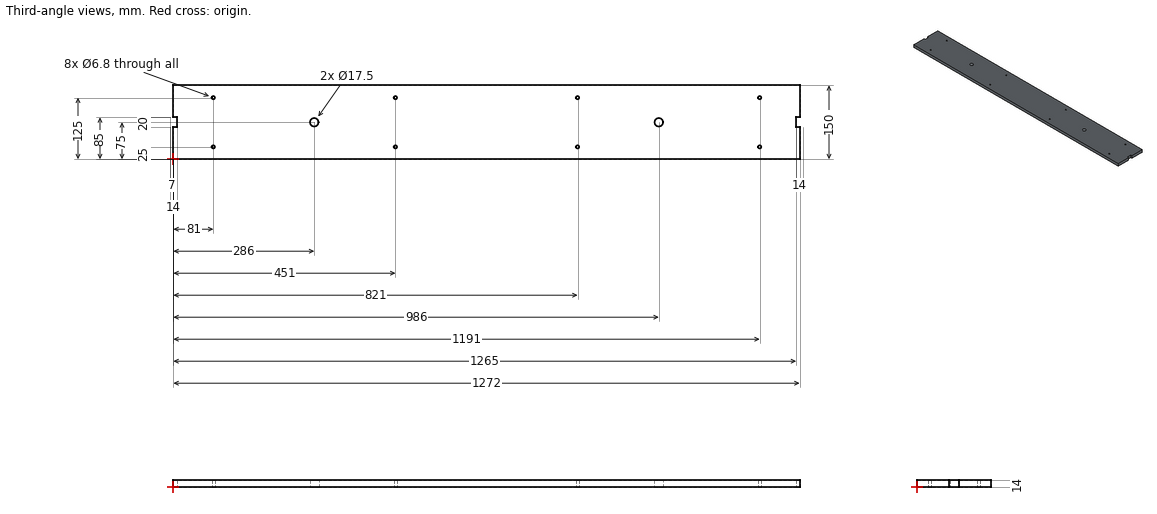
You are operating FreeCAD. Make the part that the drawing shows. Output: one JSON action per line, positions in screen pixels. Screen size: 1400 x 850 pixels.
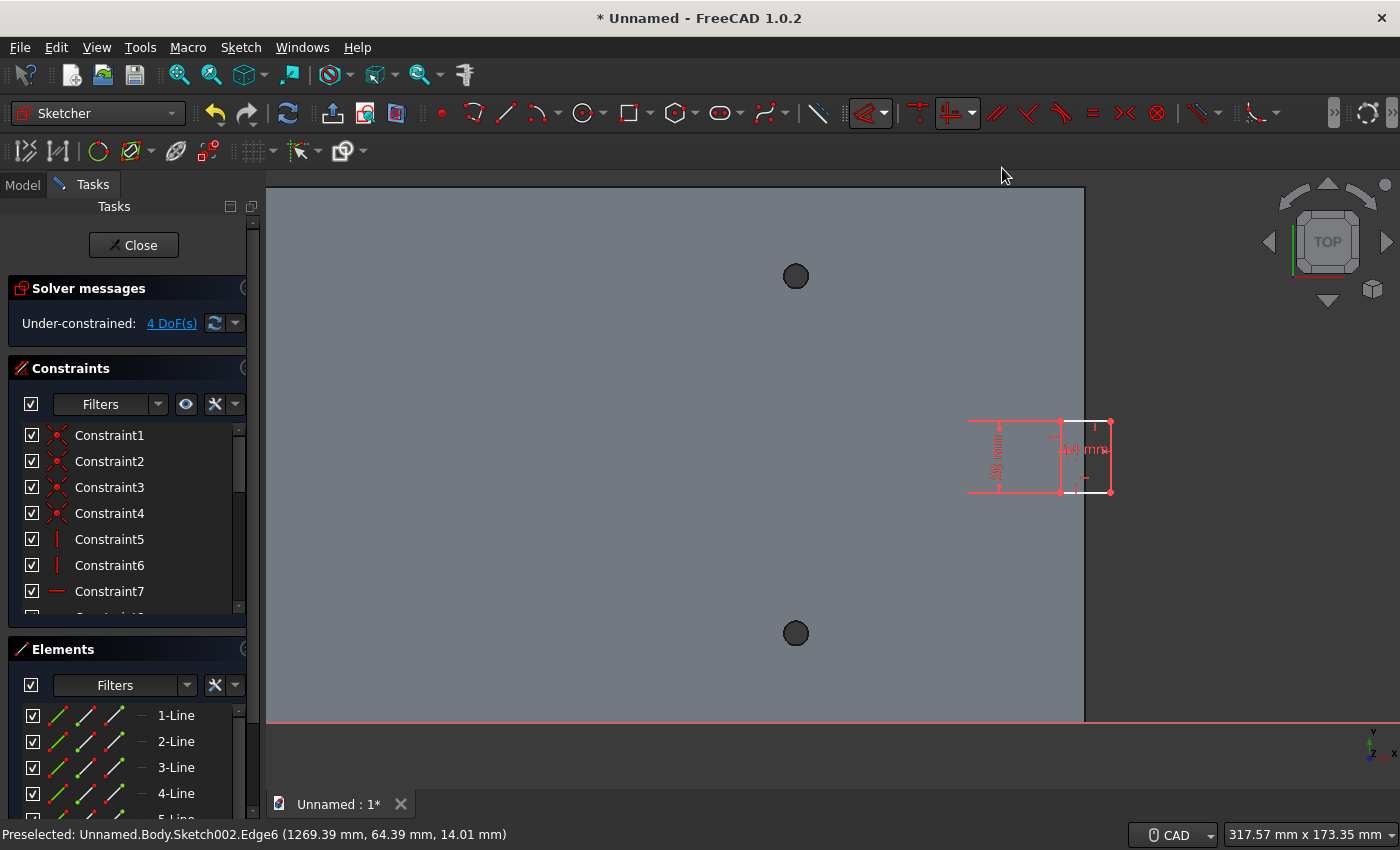
{"action": "scroll", "coordinate": [1070, 465], "scroll_direction": "down", "scroll_amount": 10}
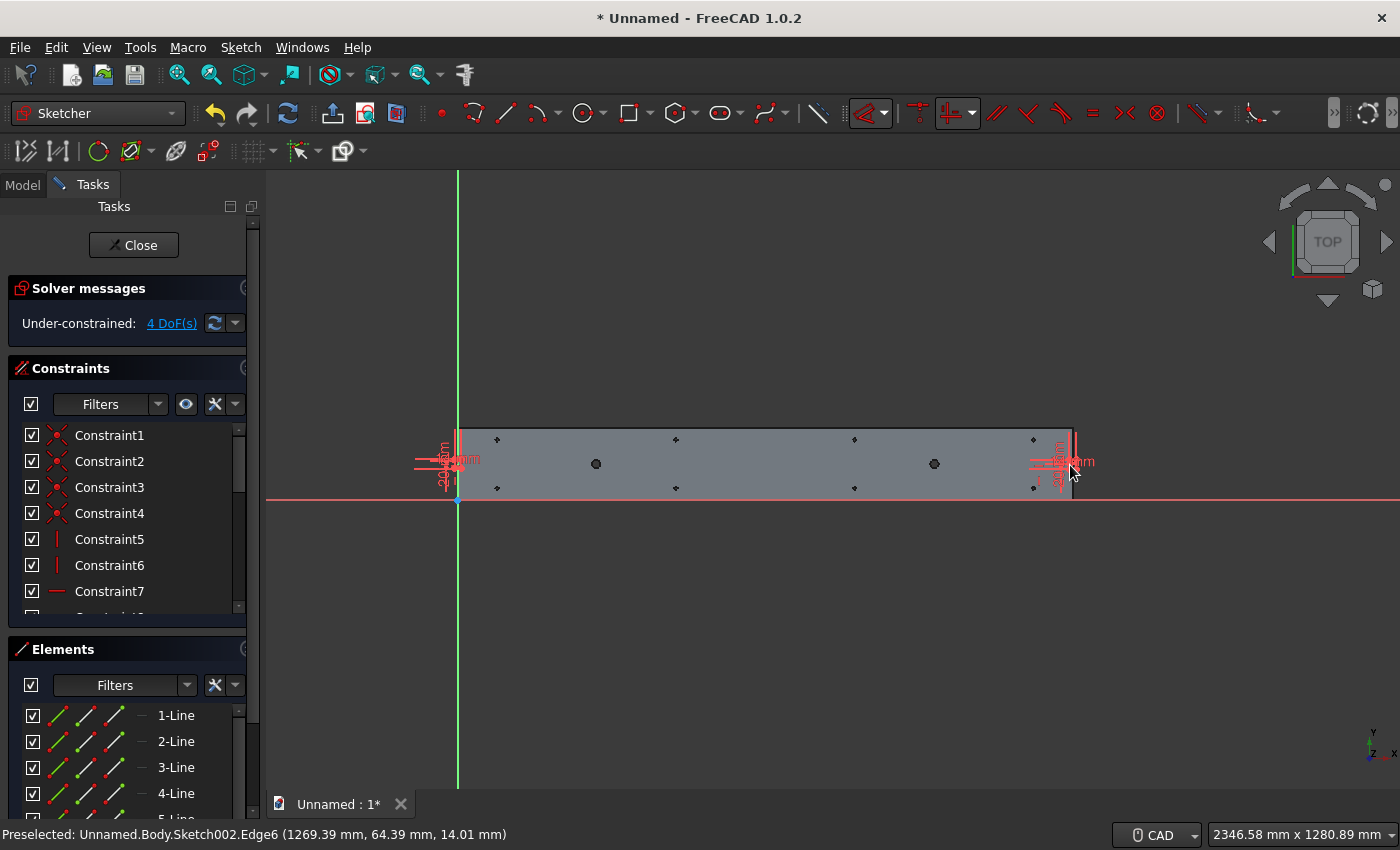
{"action": "scroll", "coordinate": [455, 459], "scroll_direction": "up", "scroll_amount": 13}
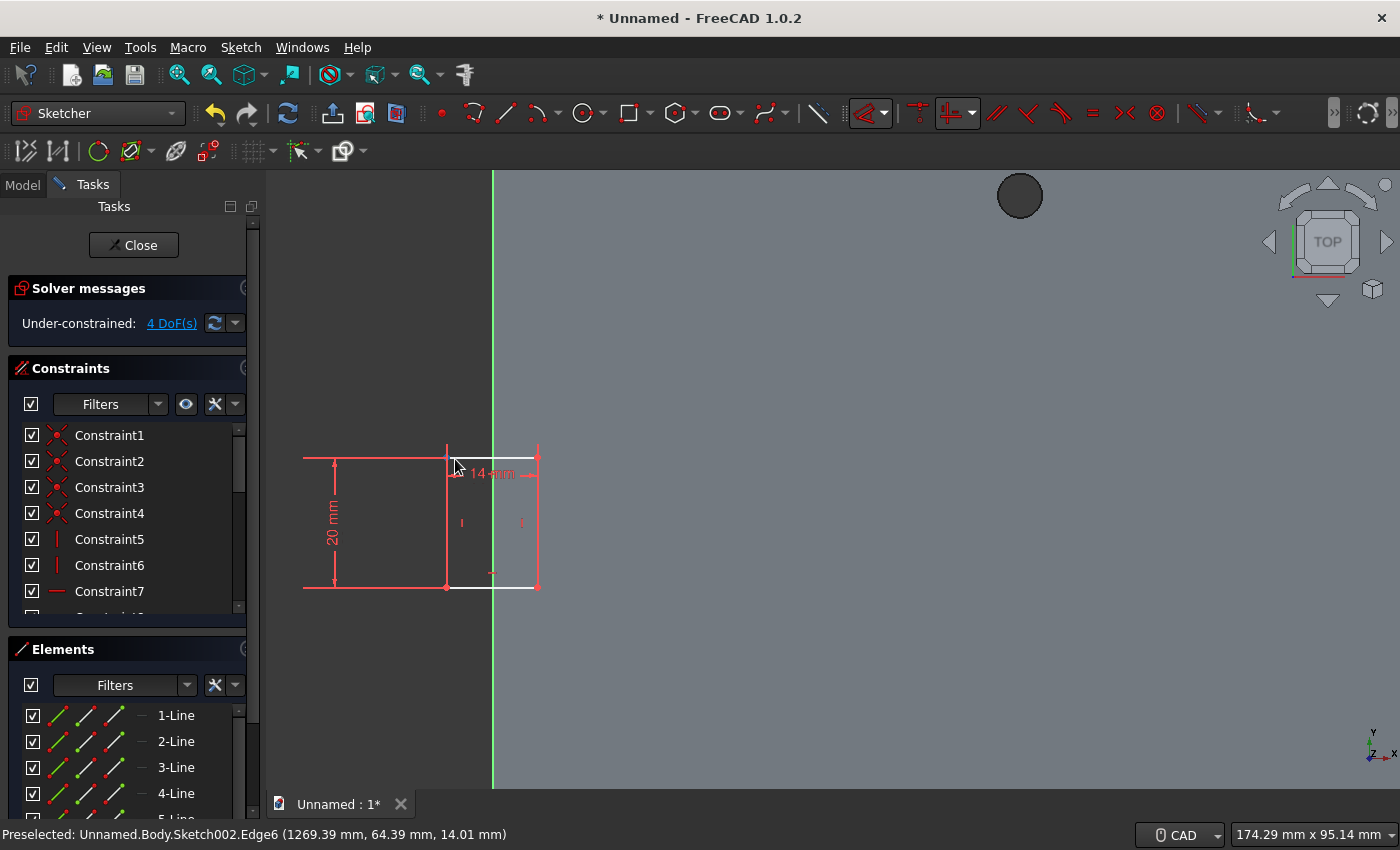
{"action": "left_click", "coordinate": [447, 458]}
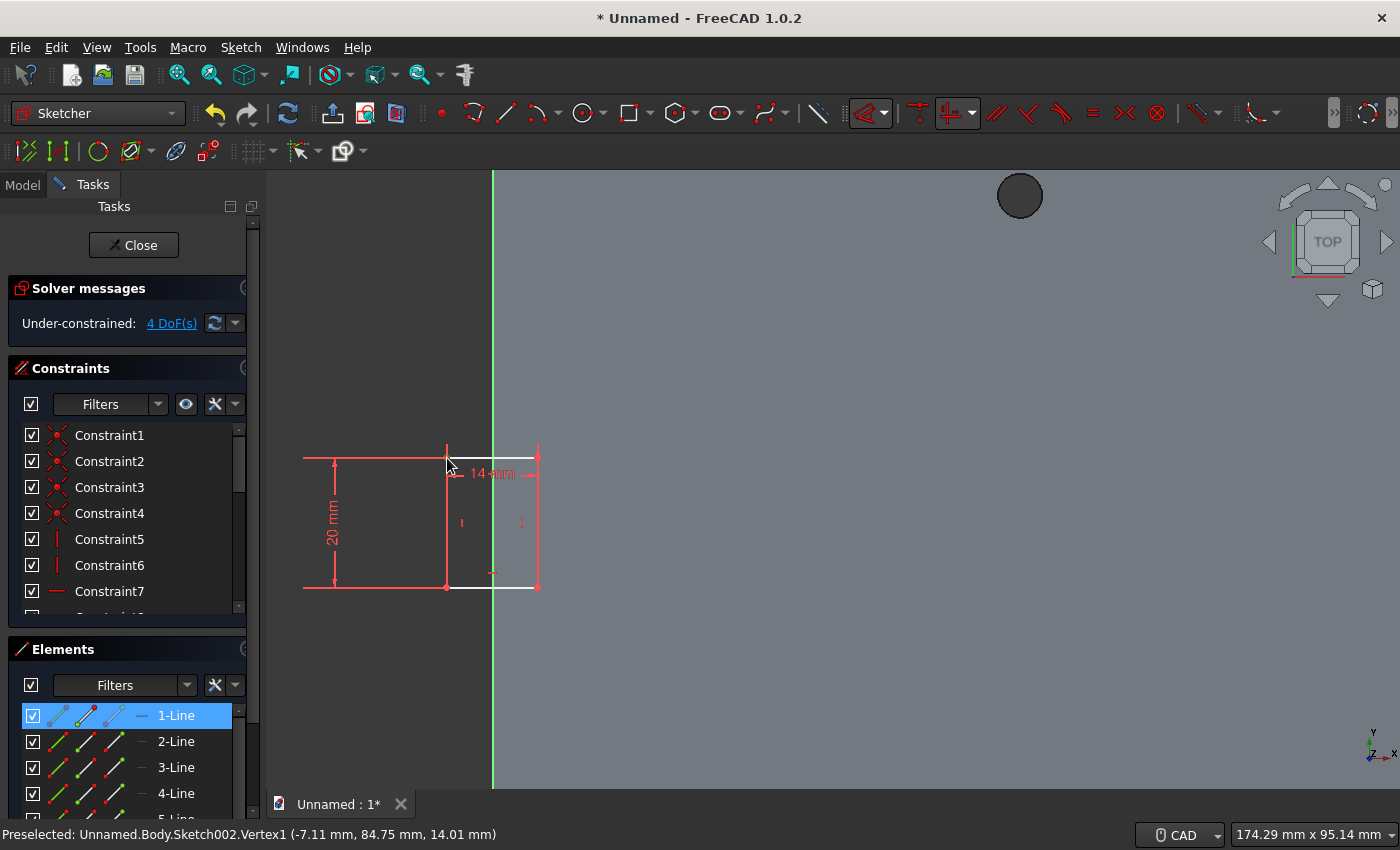
{"action": "key", "text": "l"}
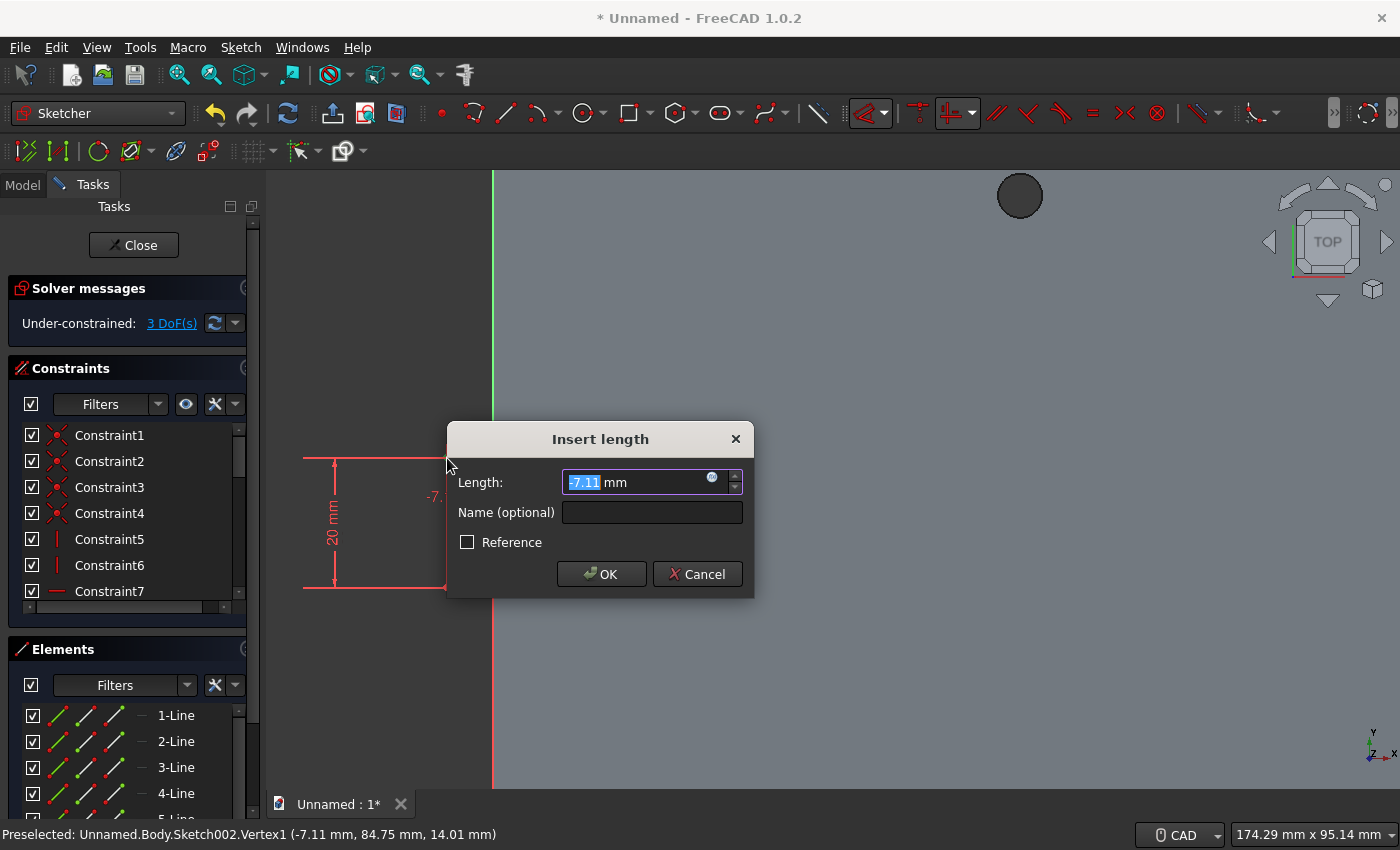
{"action": "type", "text": "-7"}
{"action": "key", "text": "Return"}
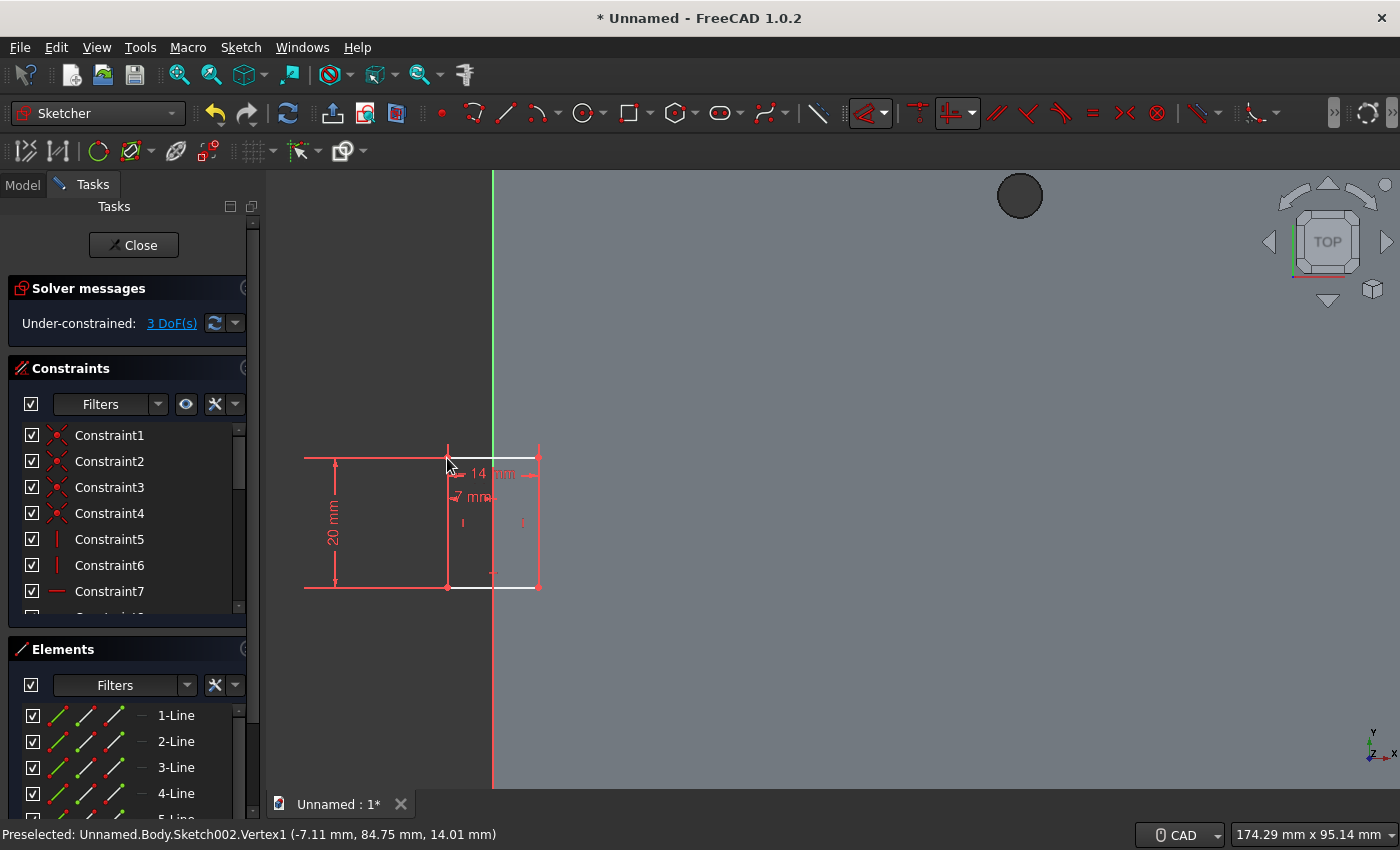
{"action": "scroll", "coordinate": [454, 459], "scroll_direction": "down", "scroll_amount": 13}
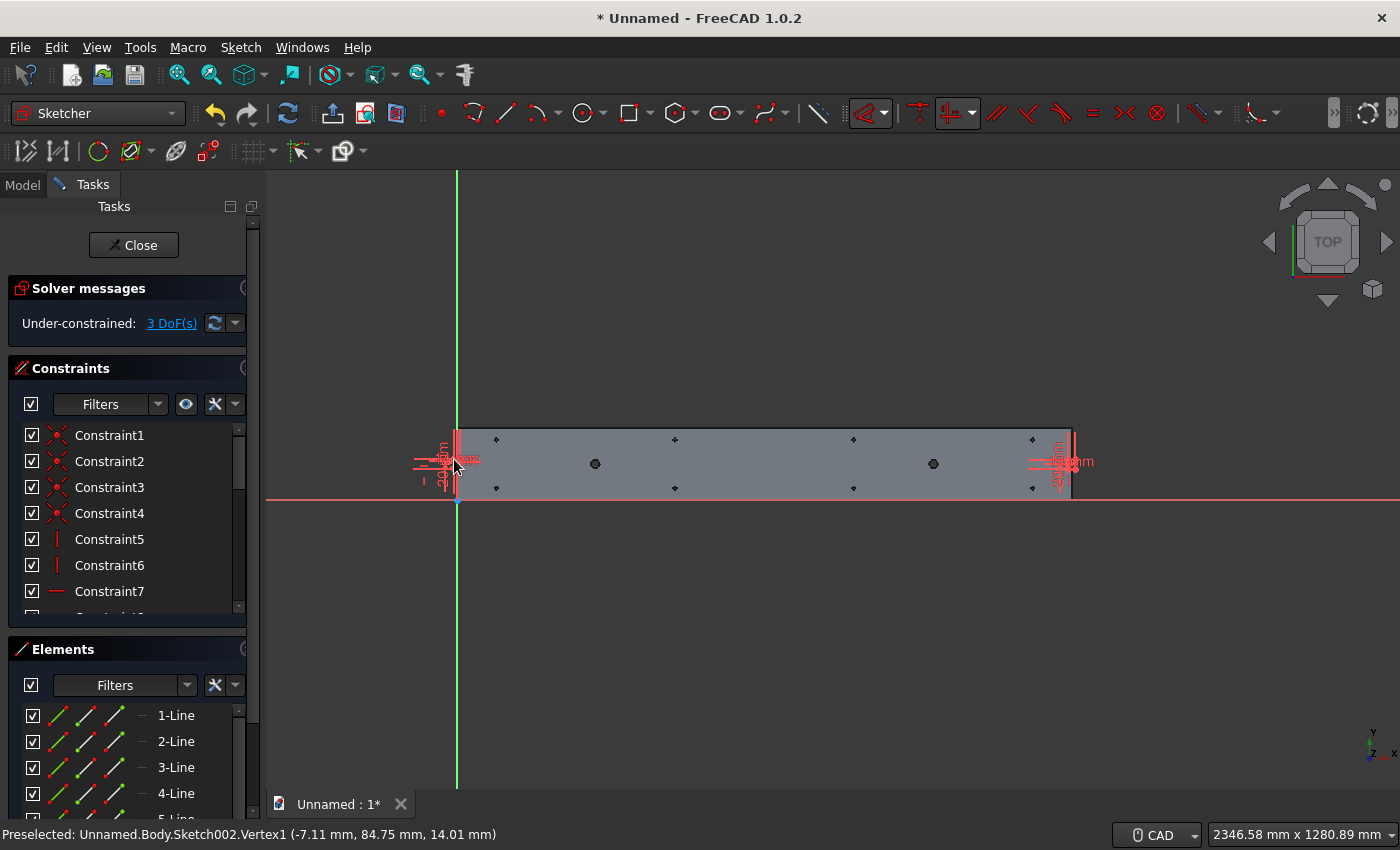
{"action": "scroll", "coordinate": [454, 459], "scroll_direction": "up", "scroll_amount": 3}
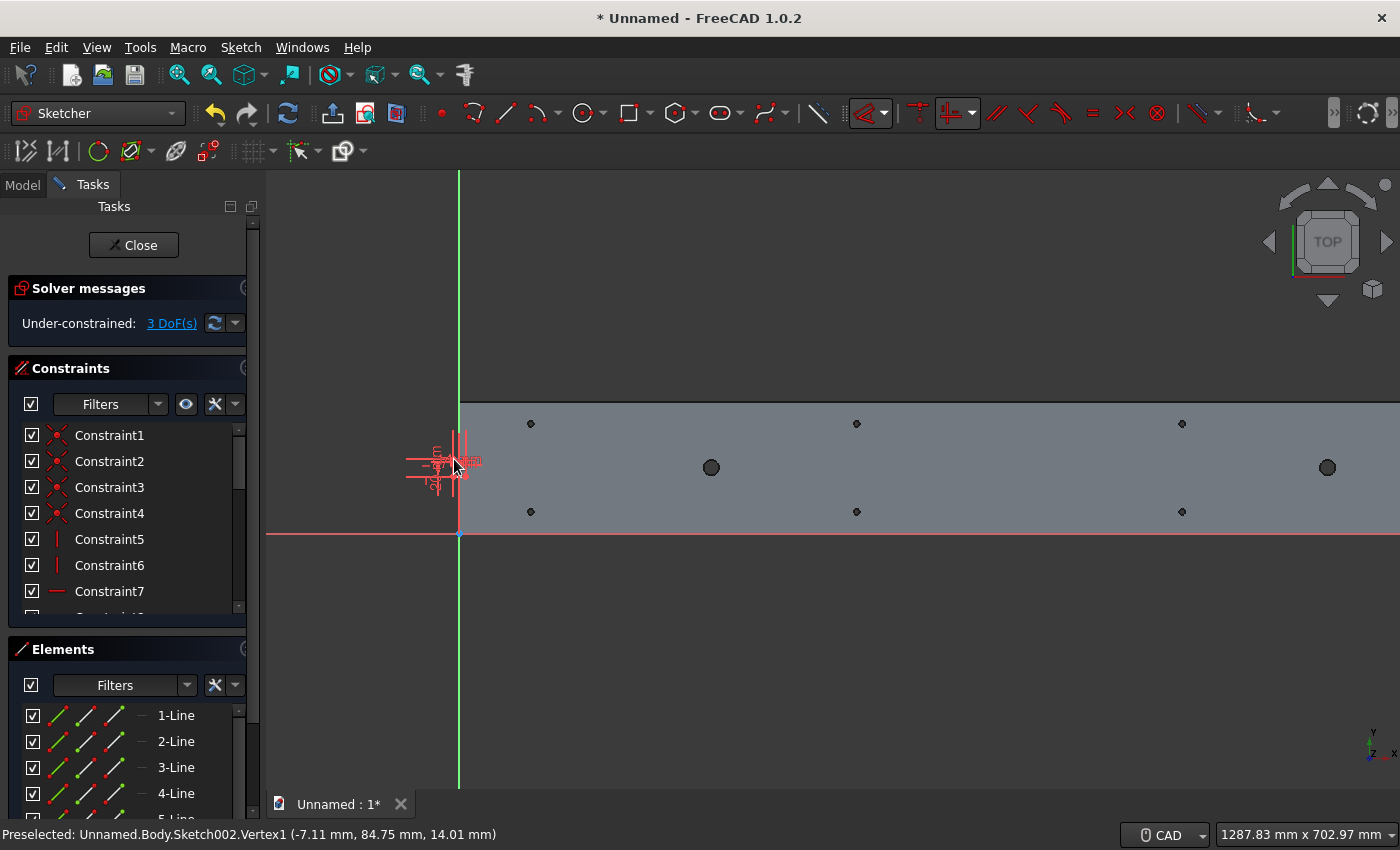
{"action": "left_click", "coordinate": [453, 459]}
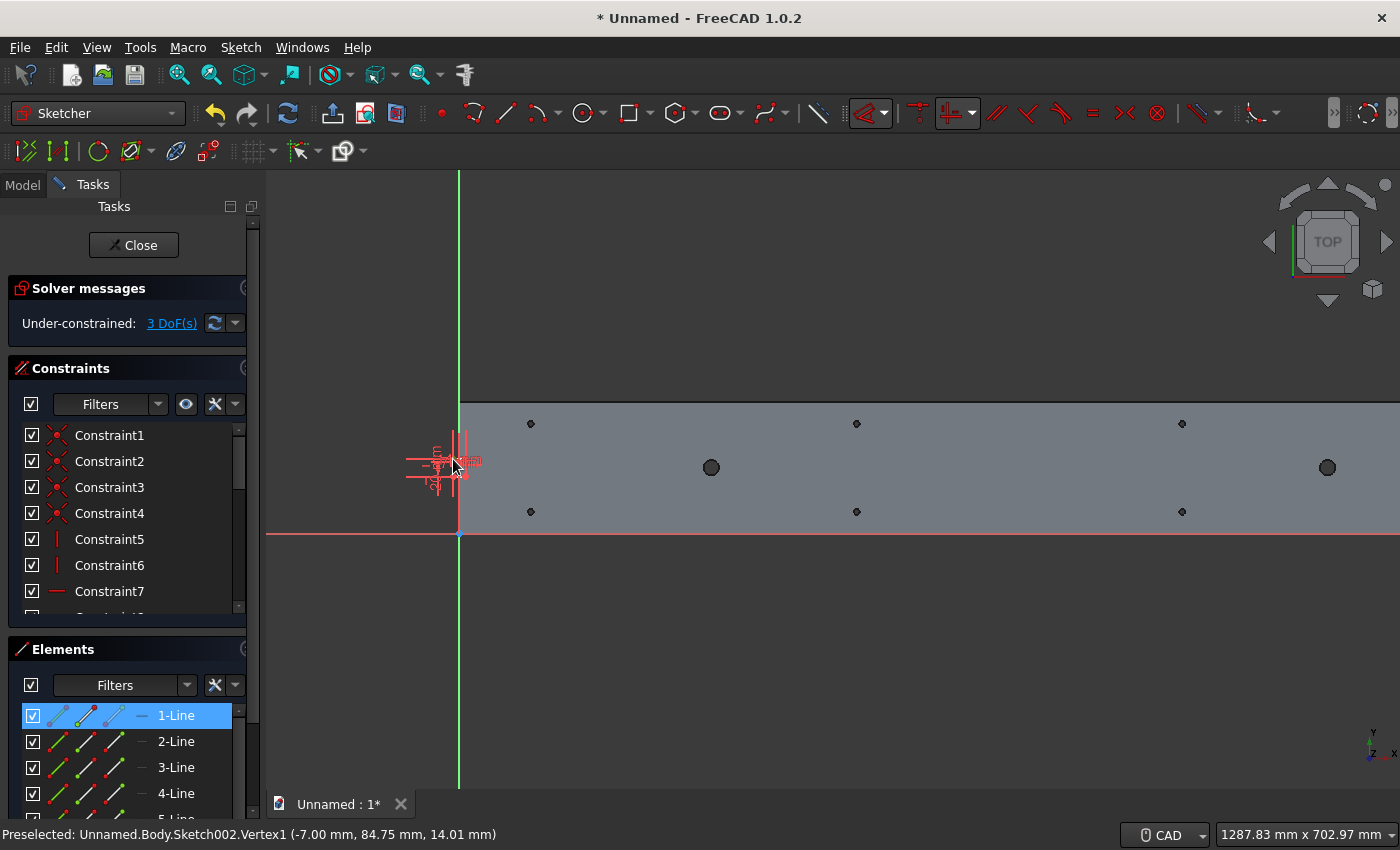
{"action": "key", "text": "i"}